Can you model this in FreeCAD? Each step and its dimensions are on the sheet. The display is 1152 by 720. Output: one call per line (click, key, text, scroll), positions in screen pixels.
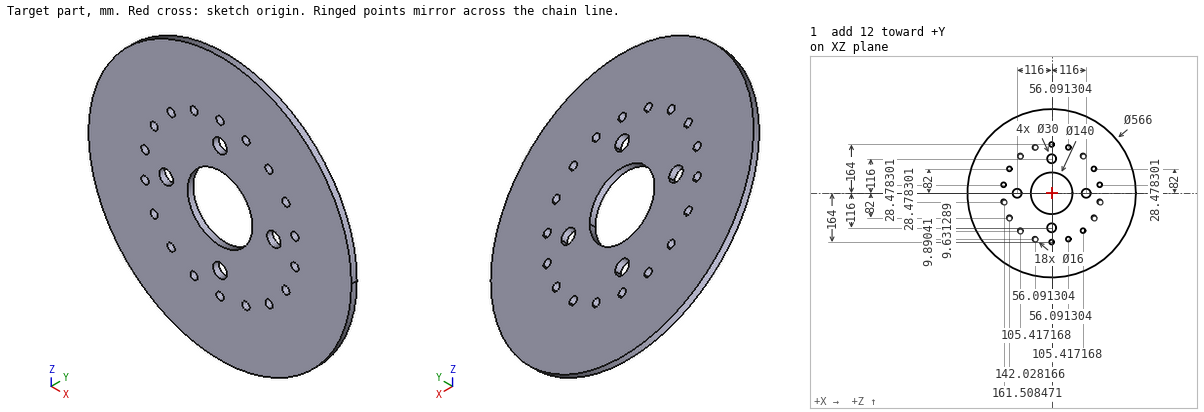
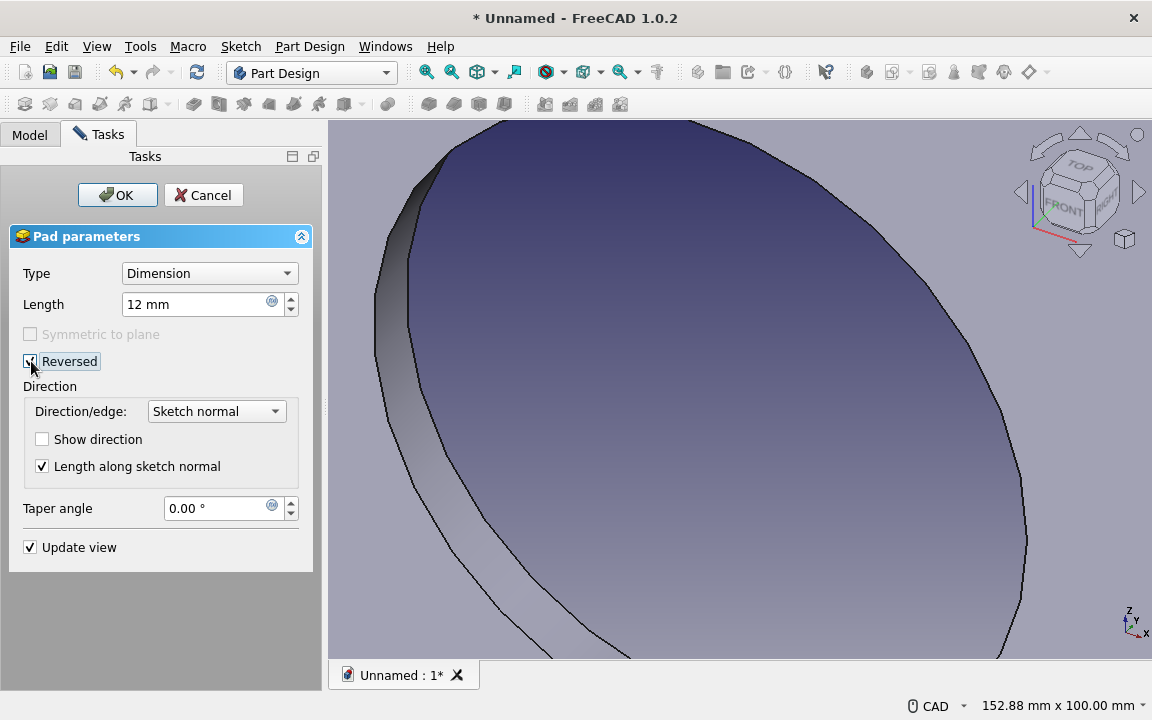
click(118, 195)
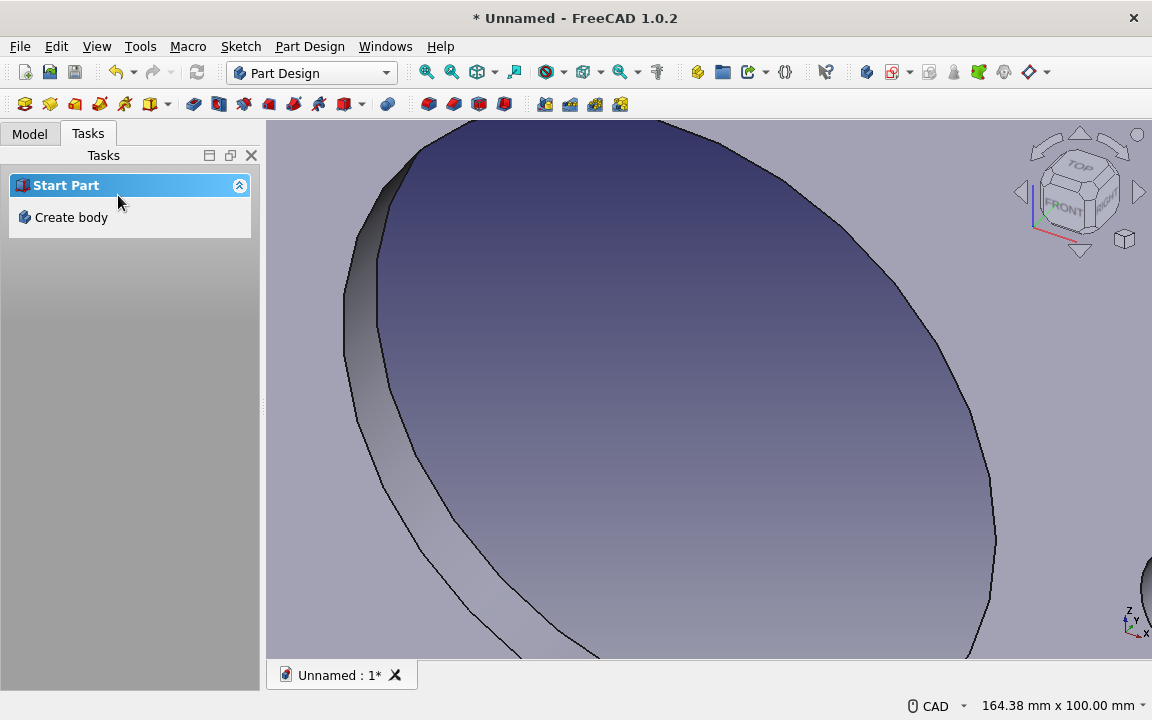
key(0)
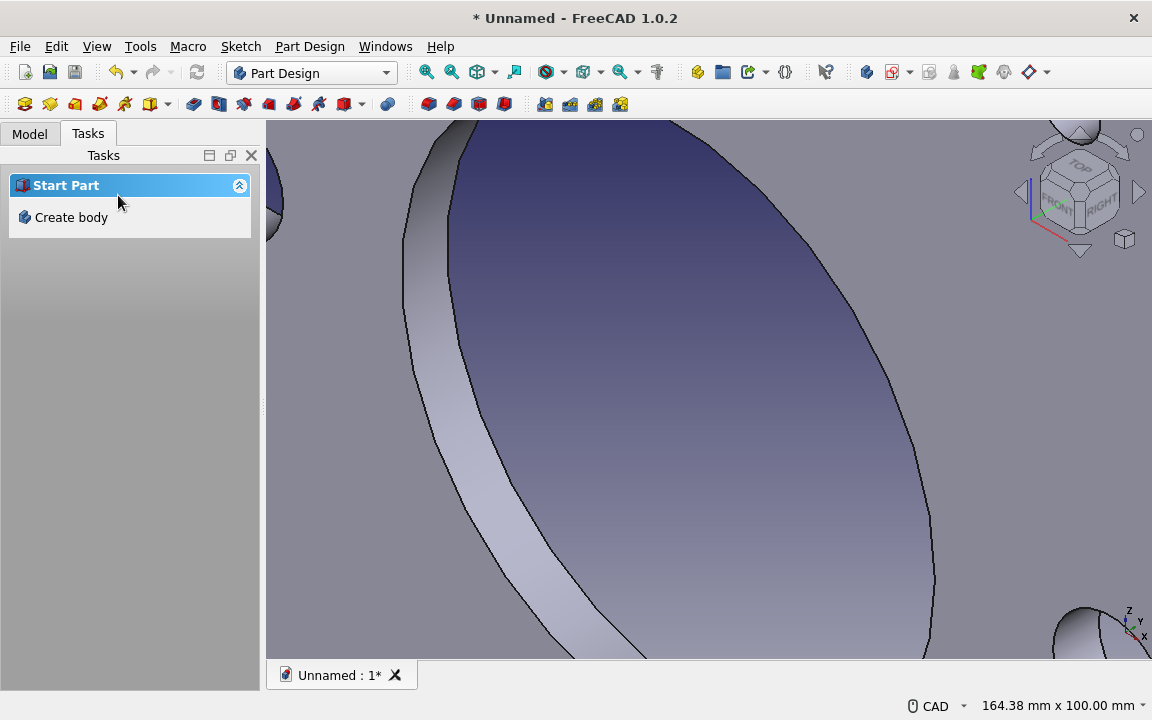
click(427, 72)